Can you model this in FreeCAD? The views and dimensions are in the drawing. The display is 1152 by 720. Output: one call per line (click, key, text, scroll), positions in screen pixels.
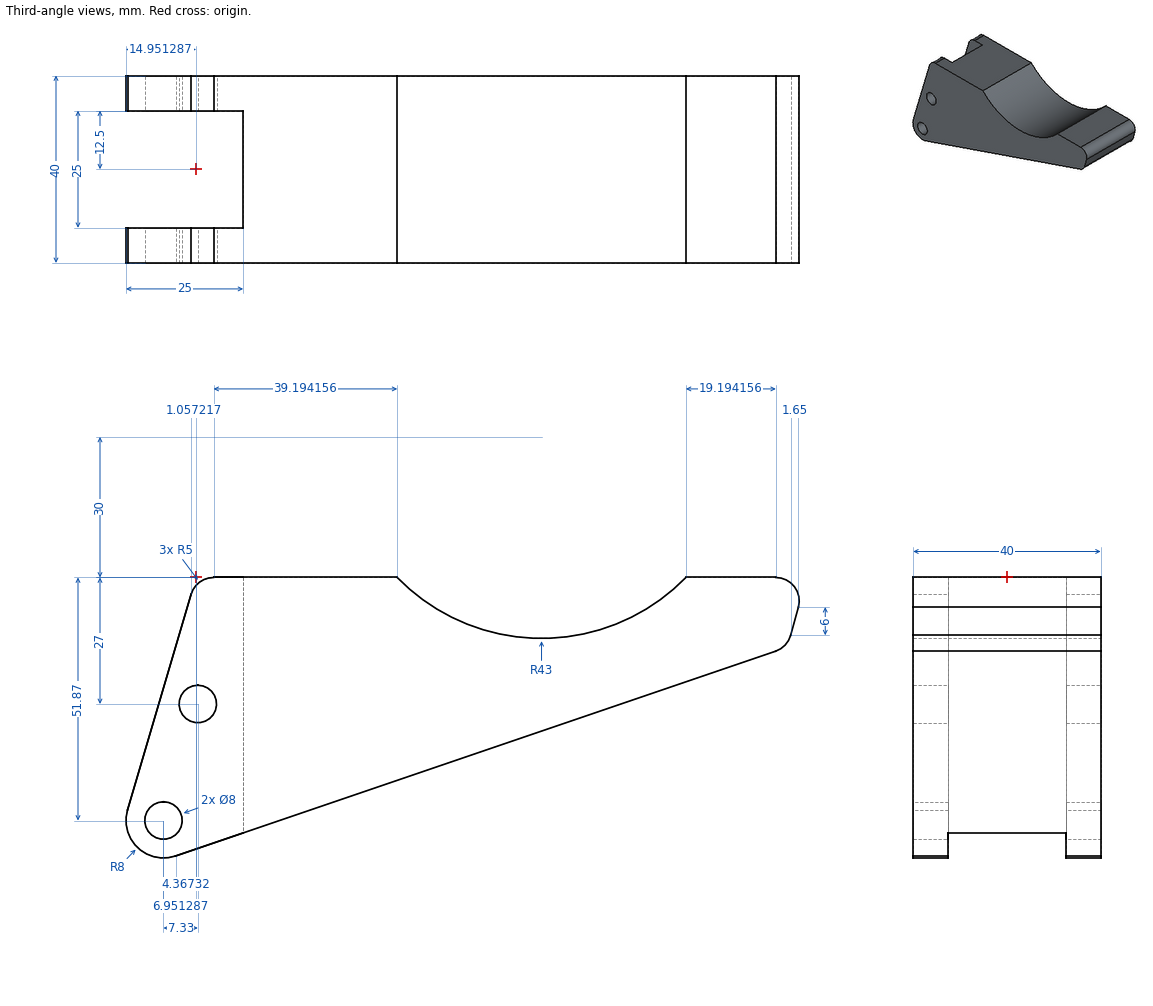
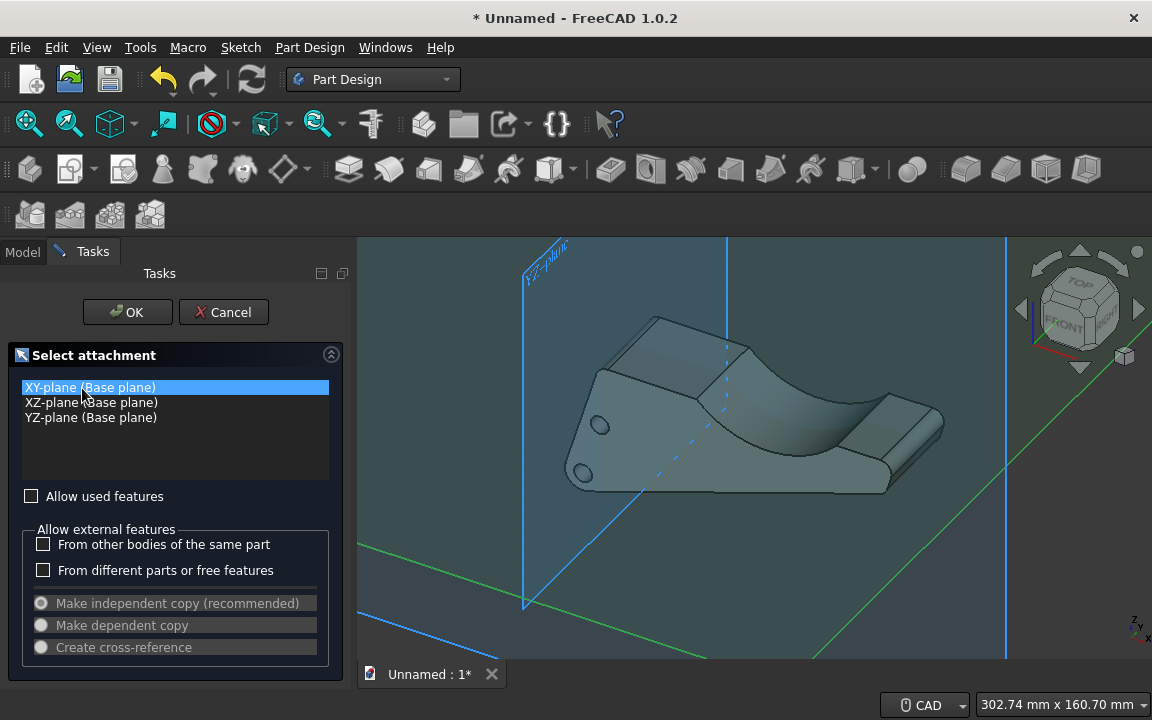
click(128, 312)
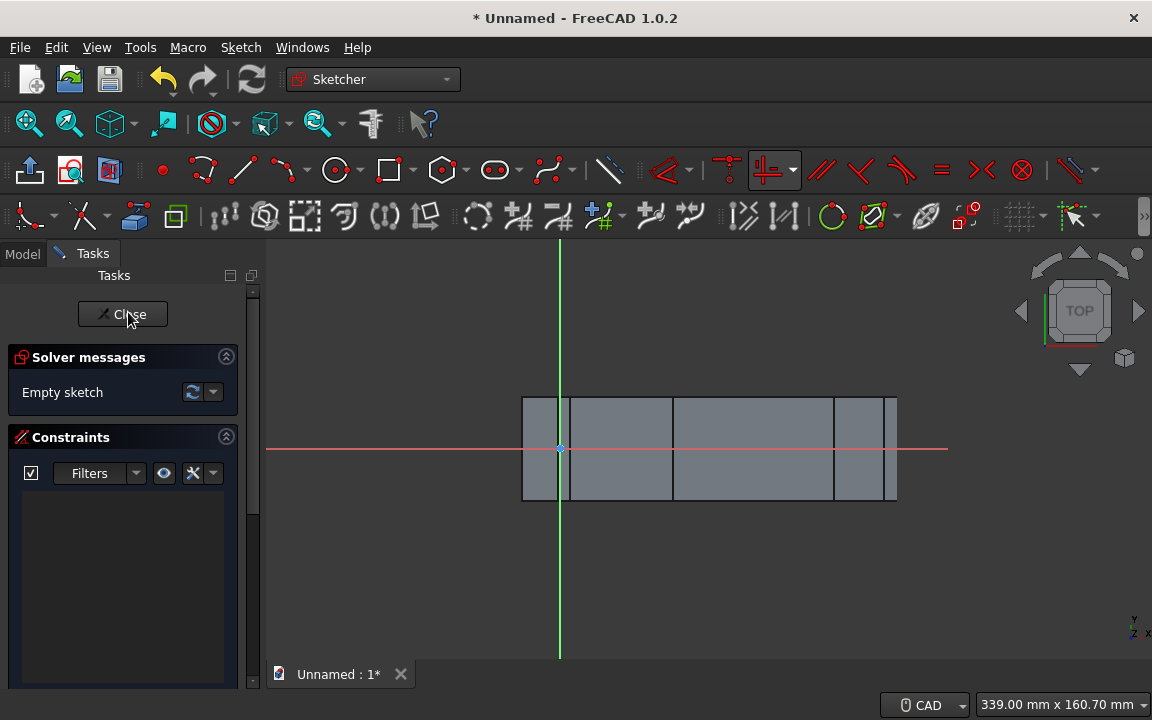
scroll(526, 449, up, 7)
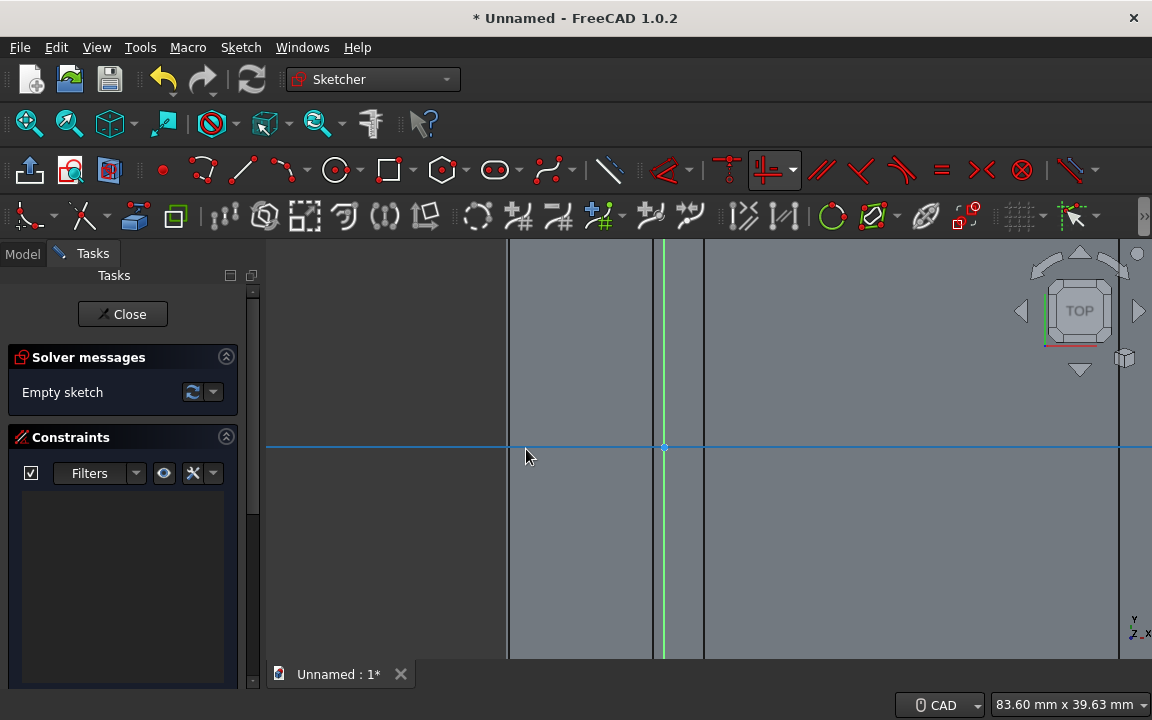
key(g)
key(r)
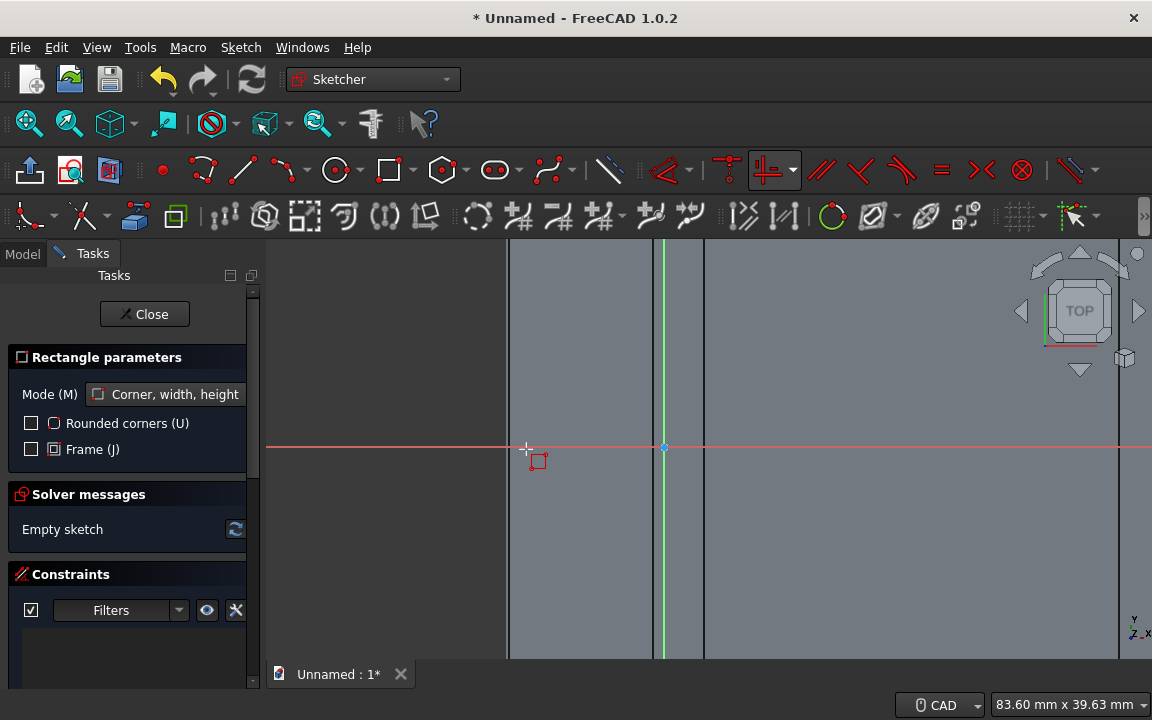
click(506, 315)
click(771, 580)
key(Escape)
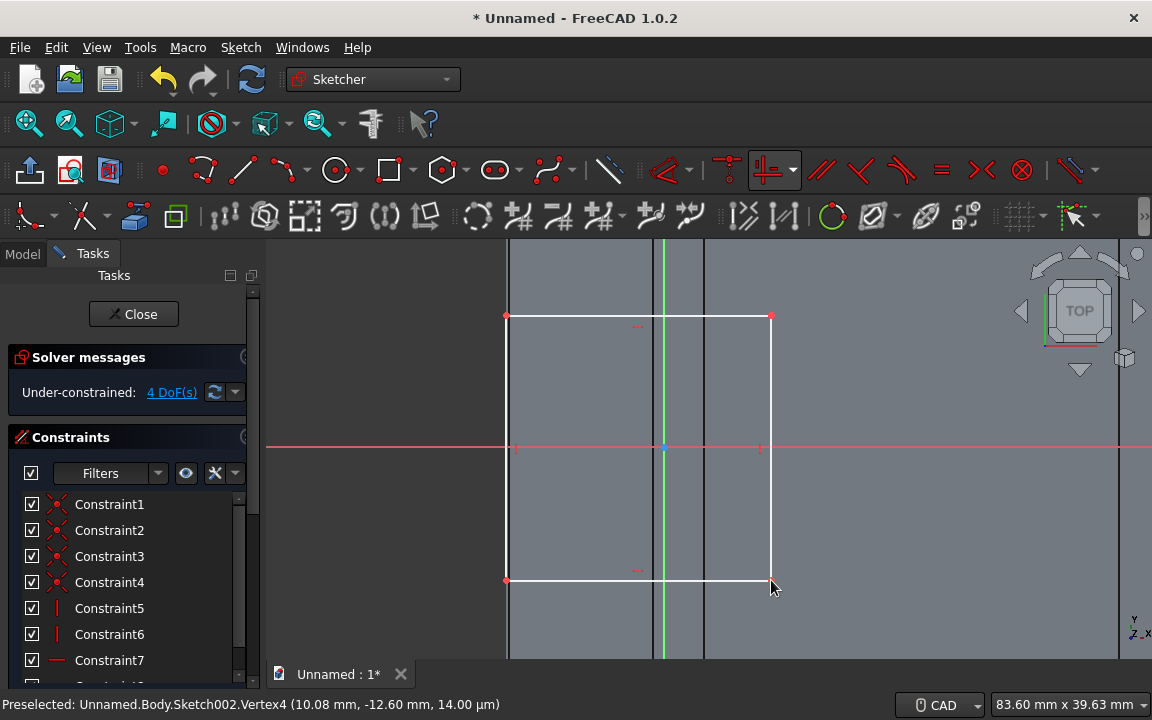
key(d)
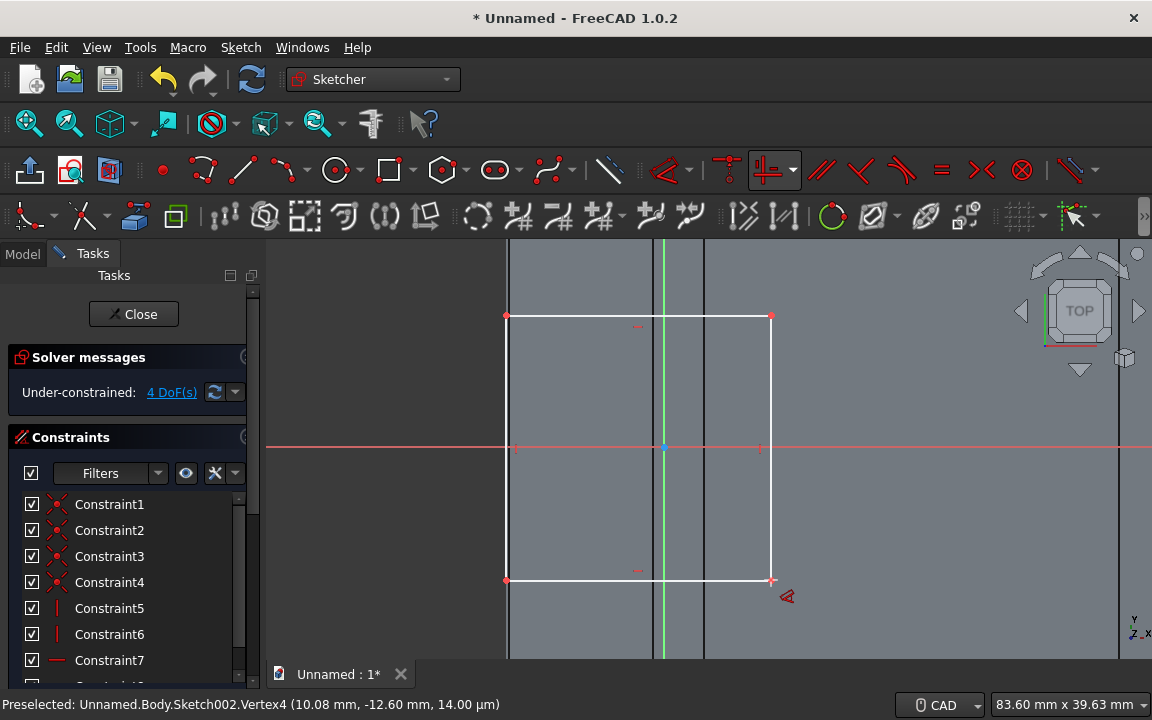
click(506, 395)
click(472, 388)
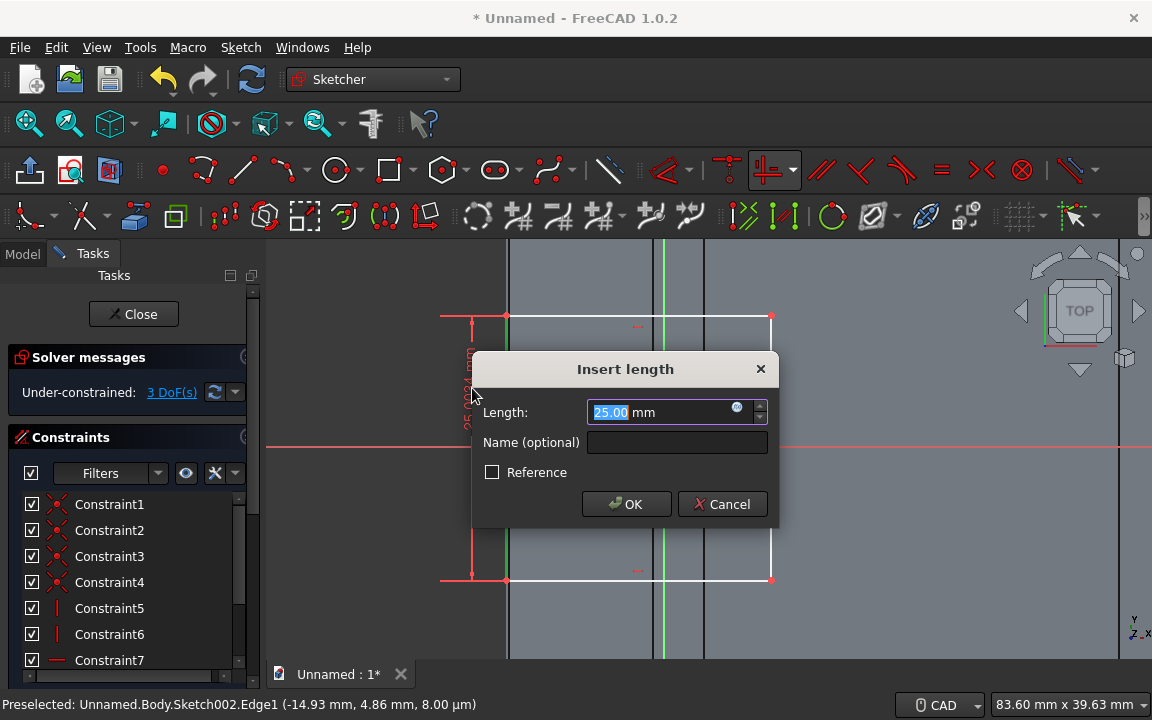
text(25)
key(Return)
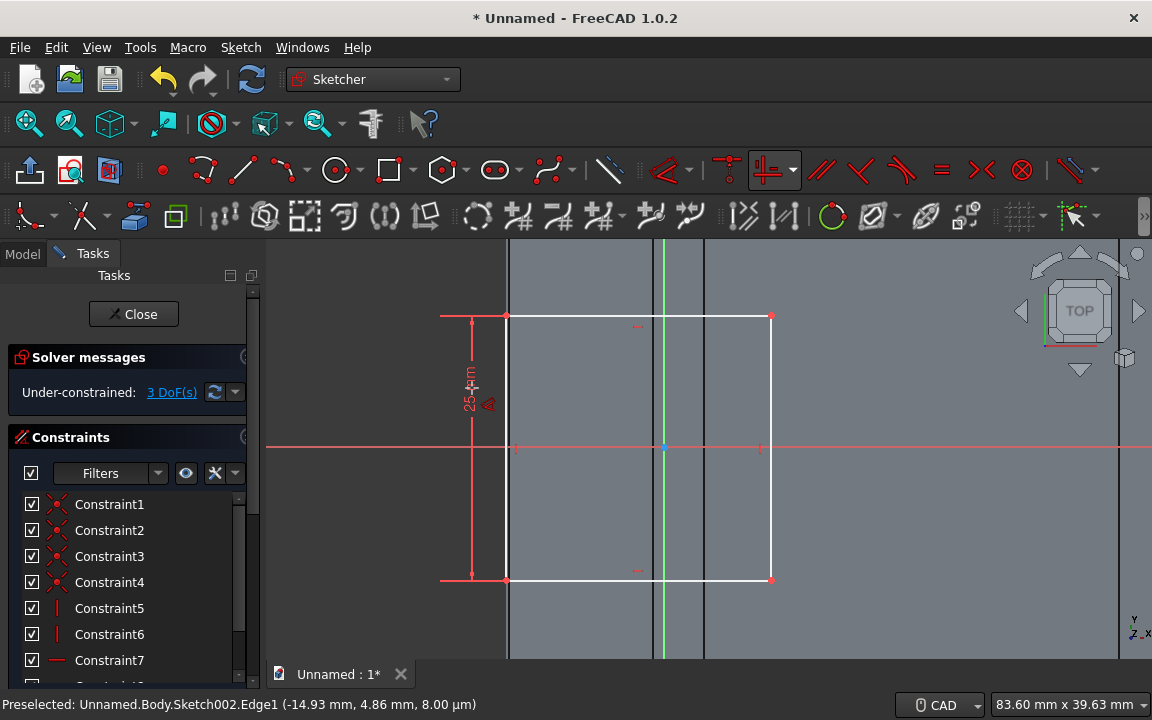
click(586, 581)
click(639, 615)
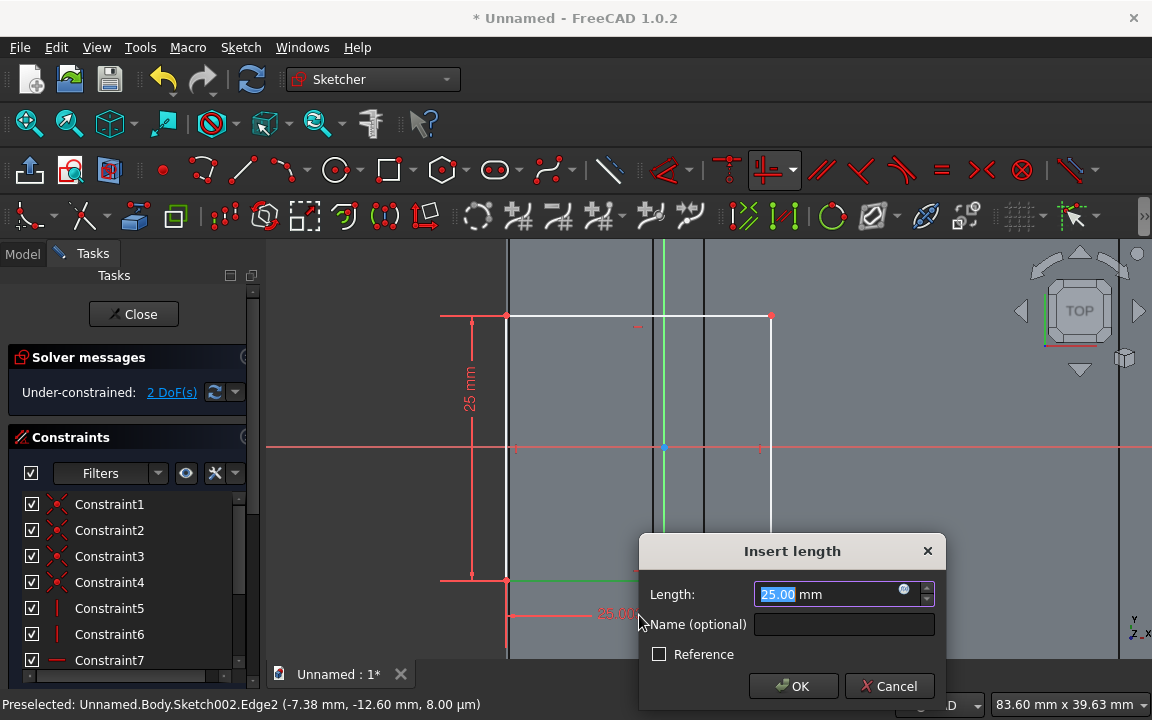
text(25)
key(Return)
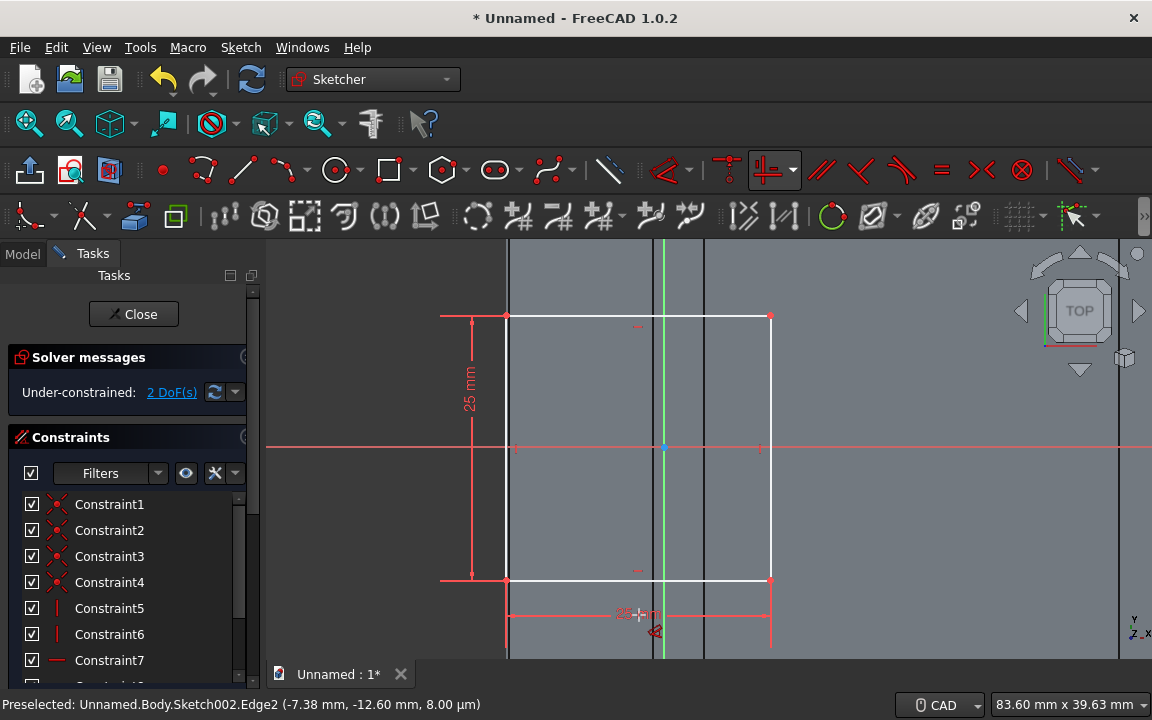
click(506, 316)
click(472, 351)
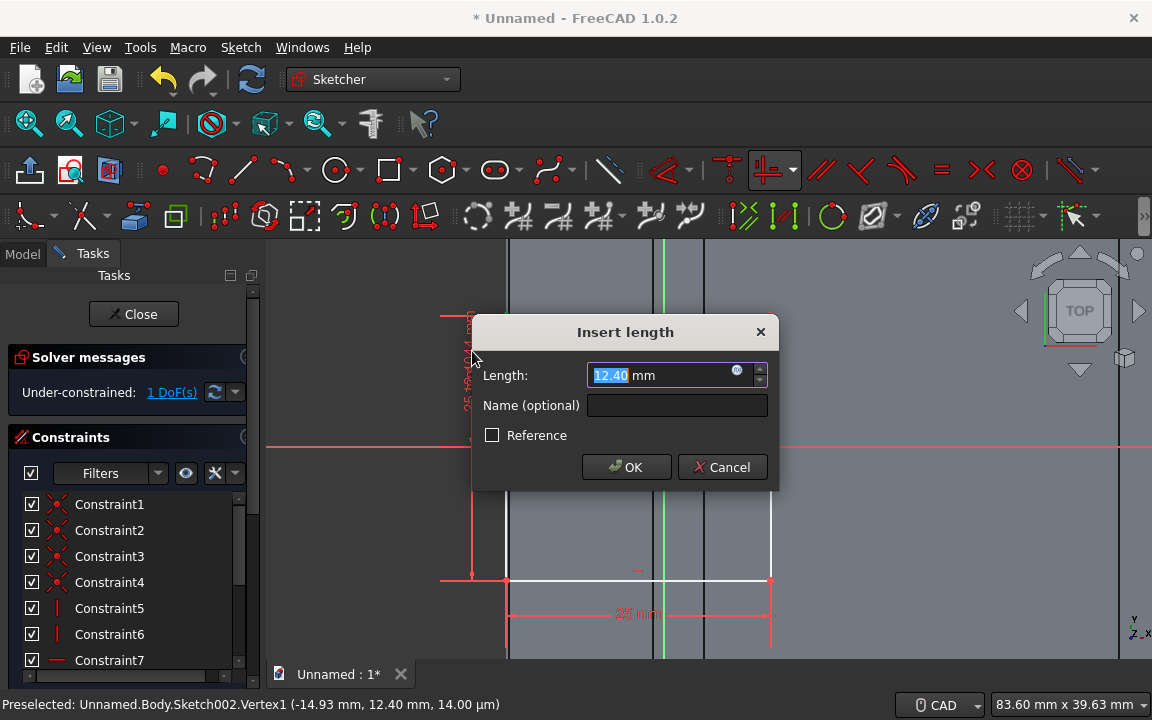
text(12.5)
key(Return)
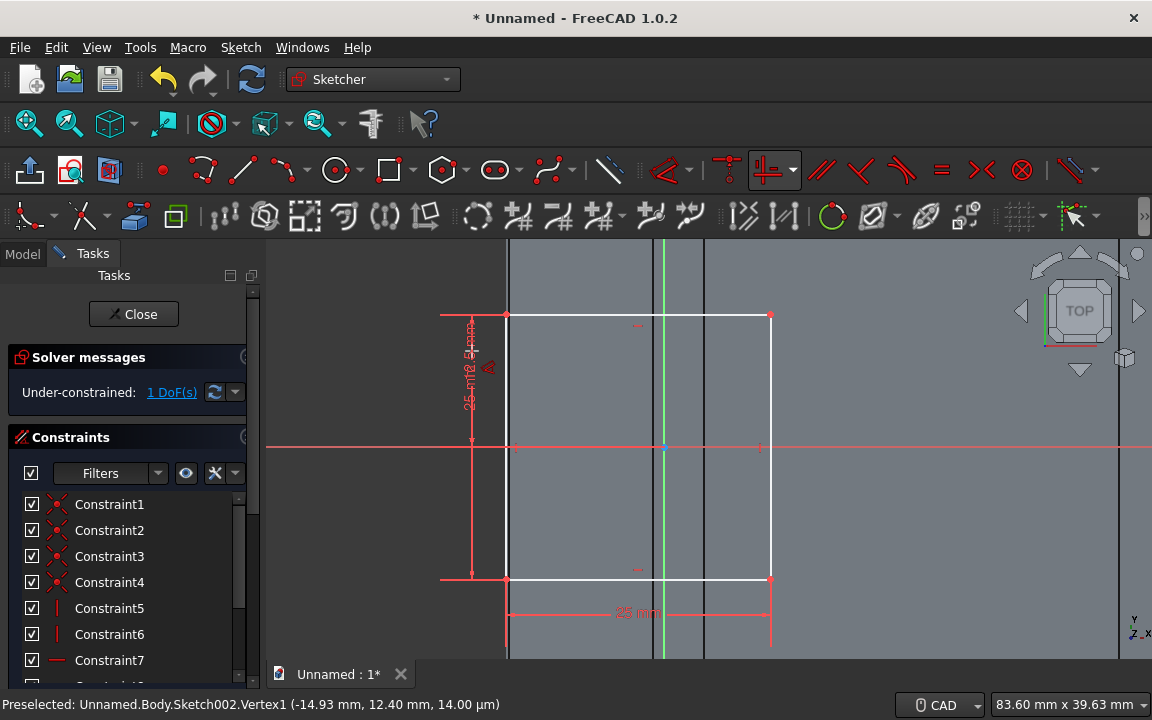
click(506, 315)
click(585, 281)